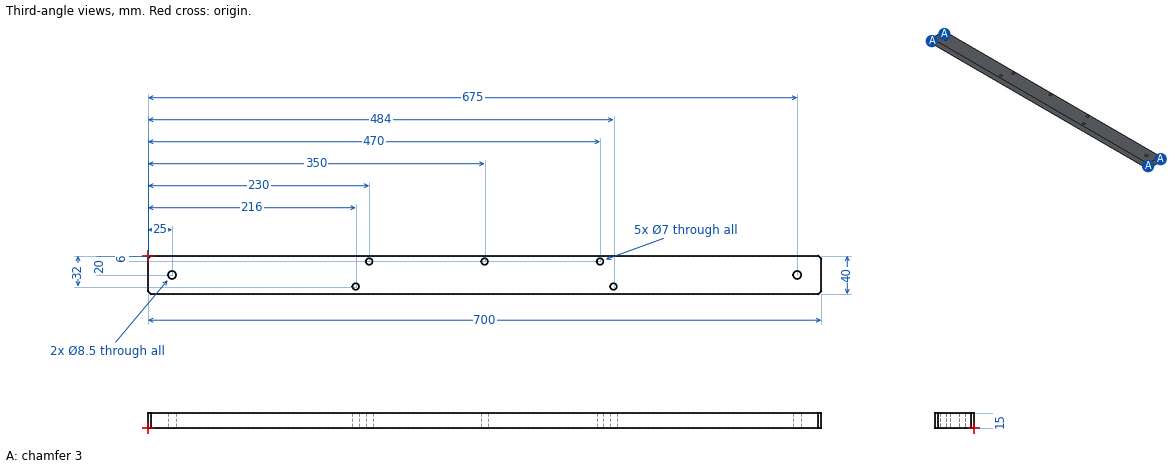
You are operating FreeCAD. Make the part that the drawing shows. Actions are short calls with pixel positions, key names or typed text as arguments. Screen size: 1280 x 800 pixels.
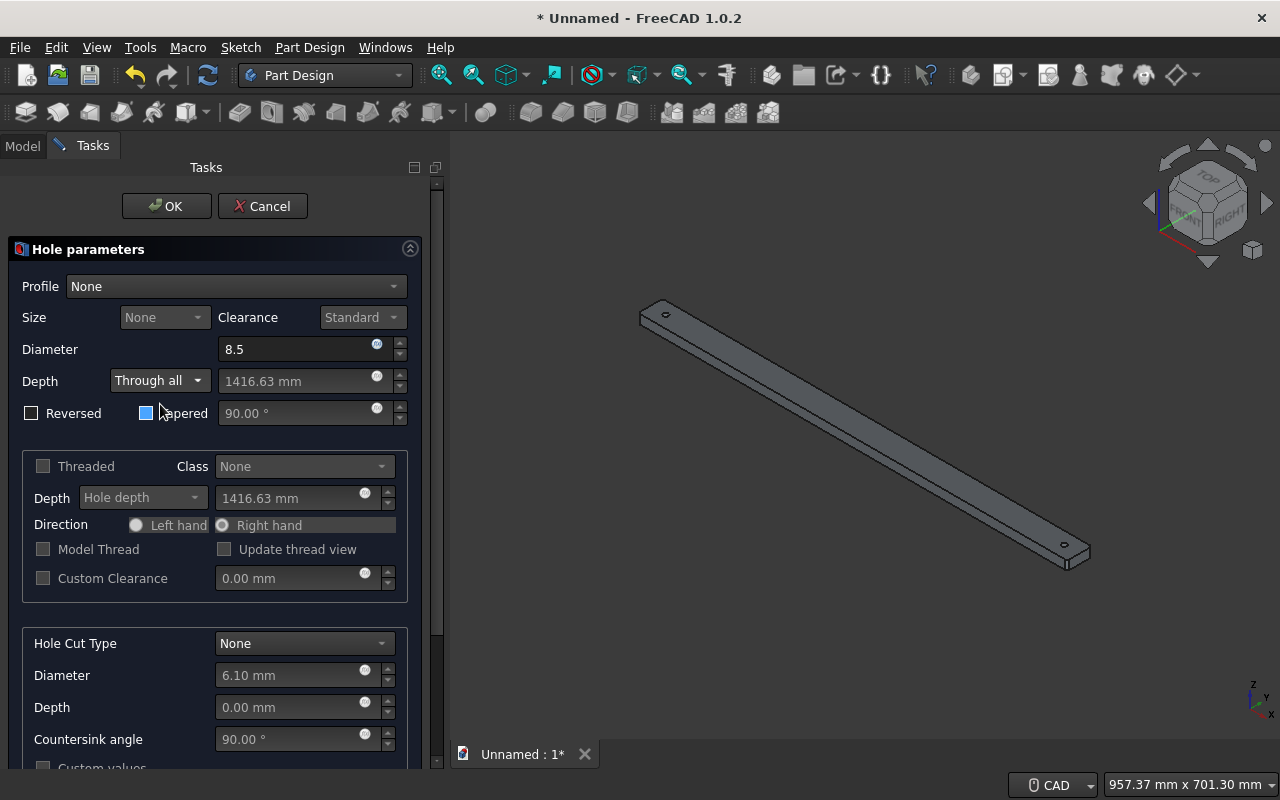
click(167, 206)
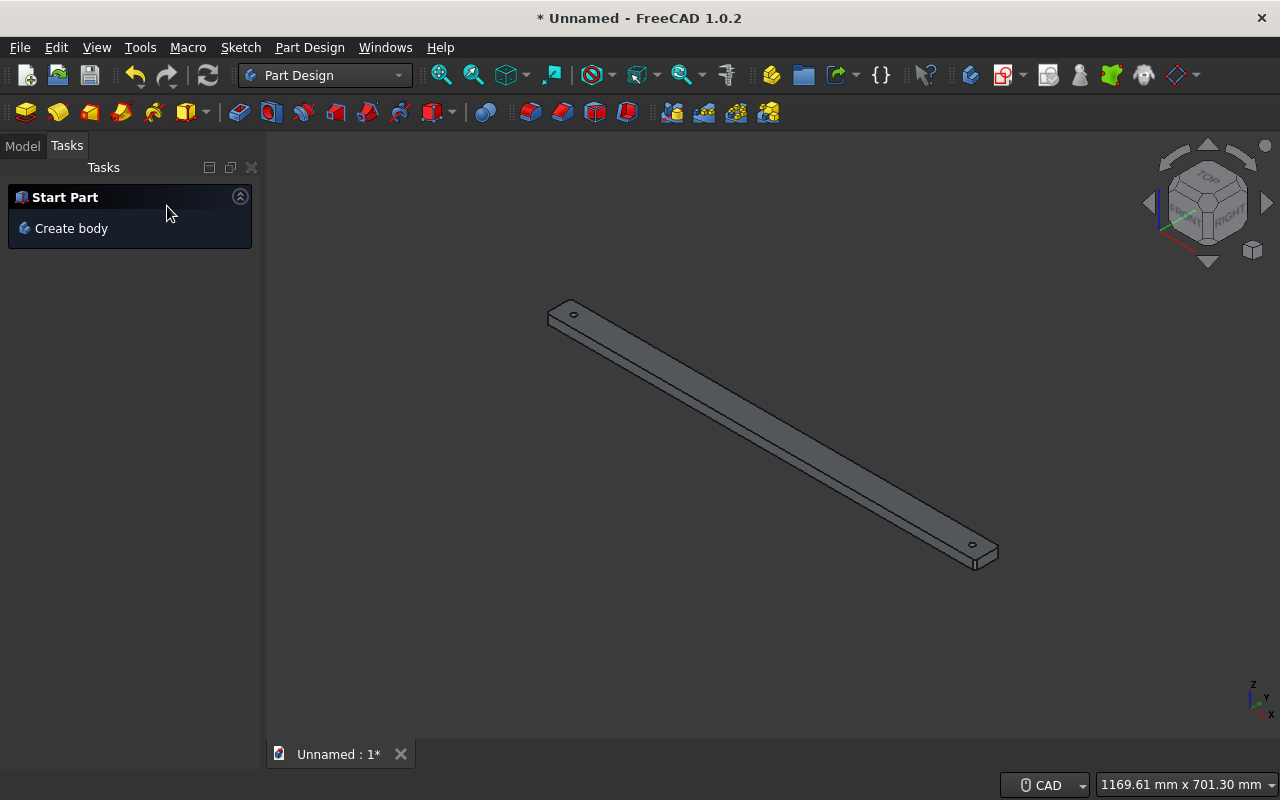
click(442, 76)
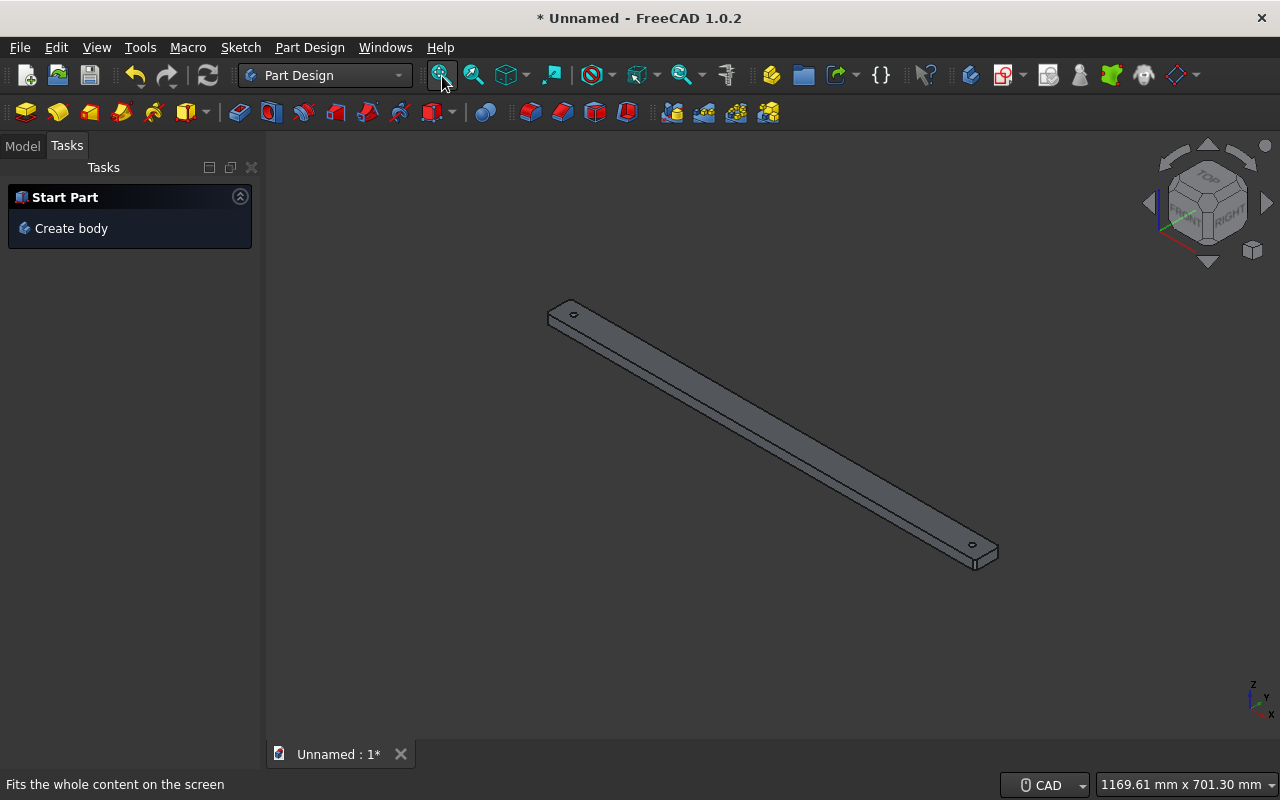
click(957, 535)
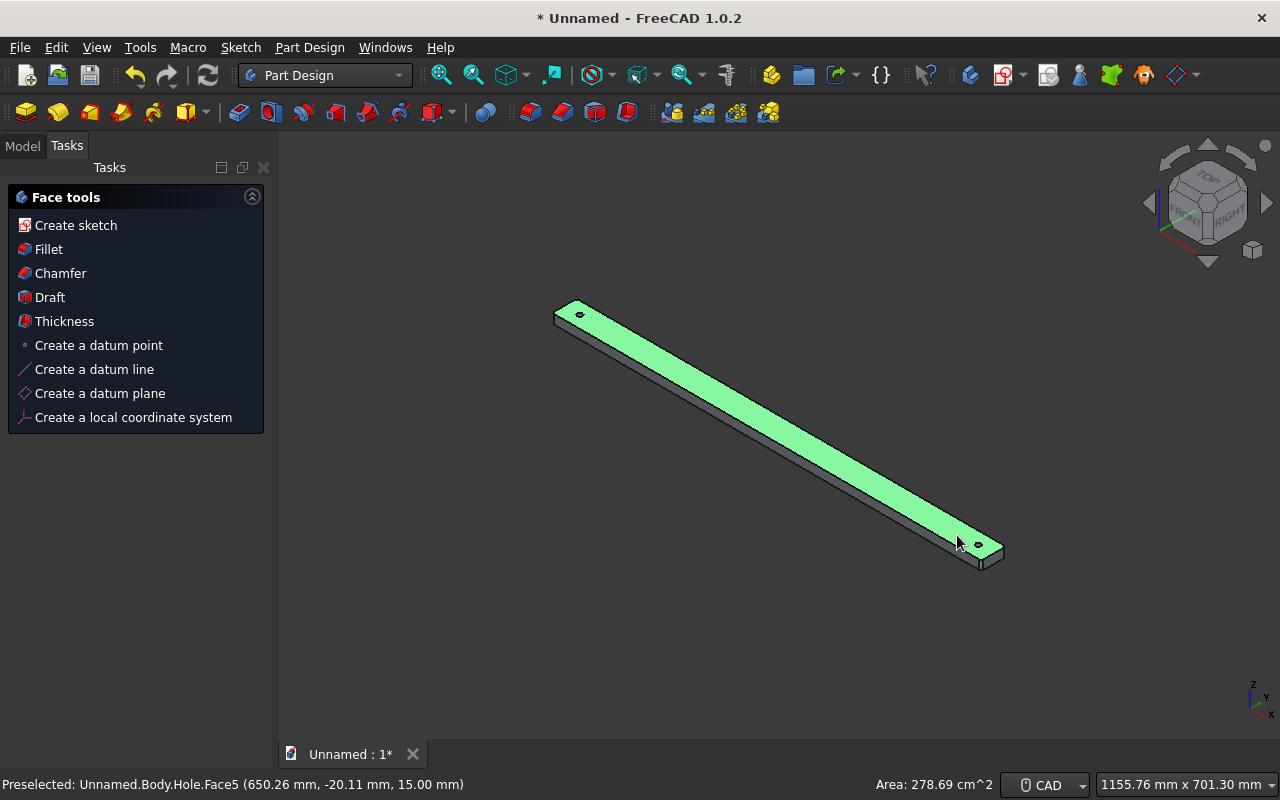
click(1004, 76)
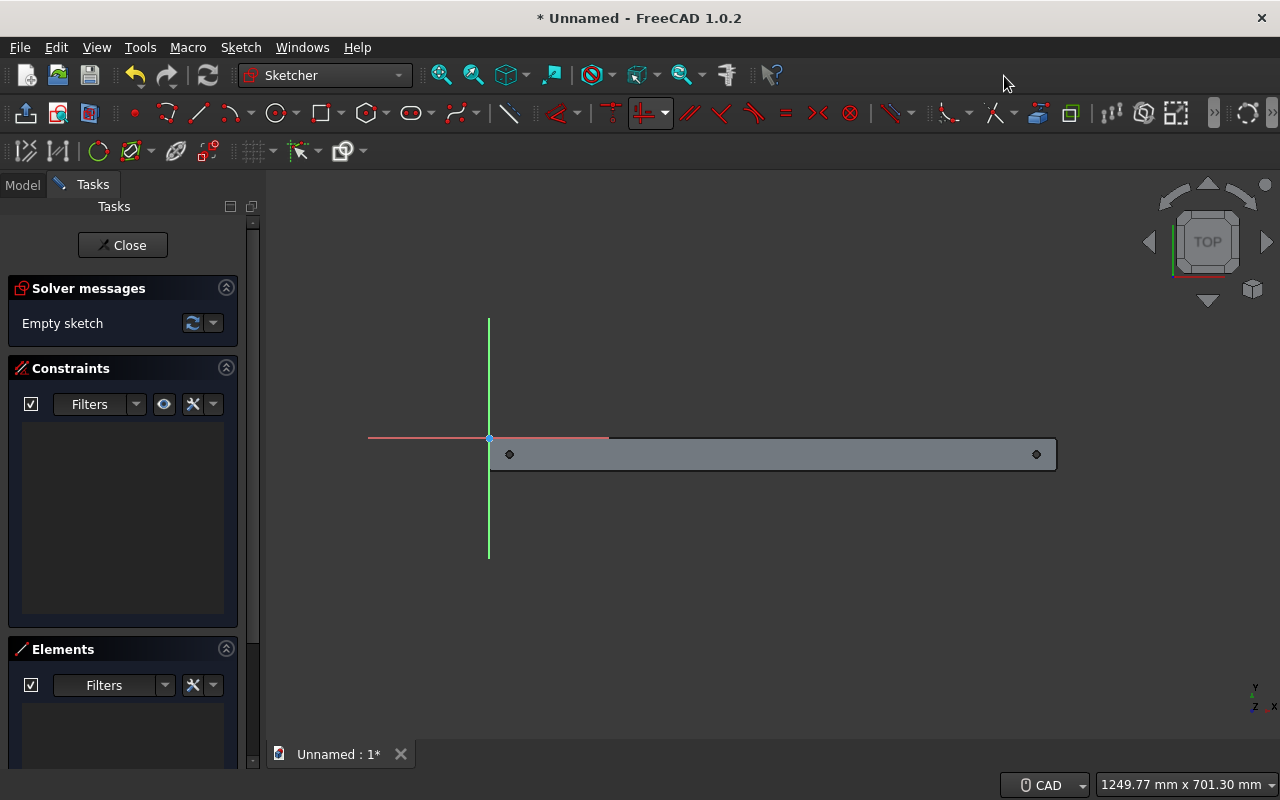
scroll(651, 449, up, 2)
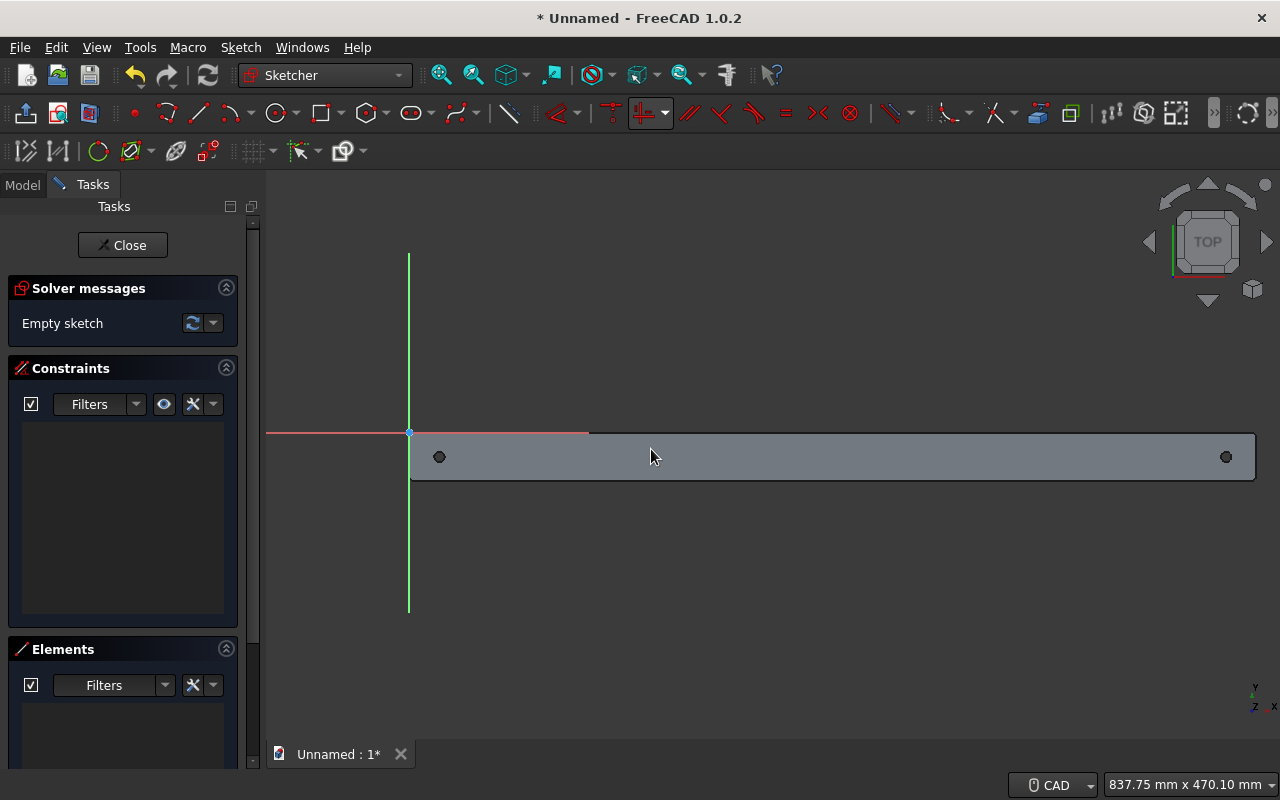
click(276, 114)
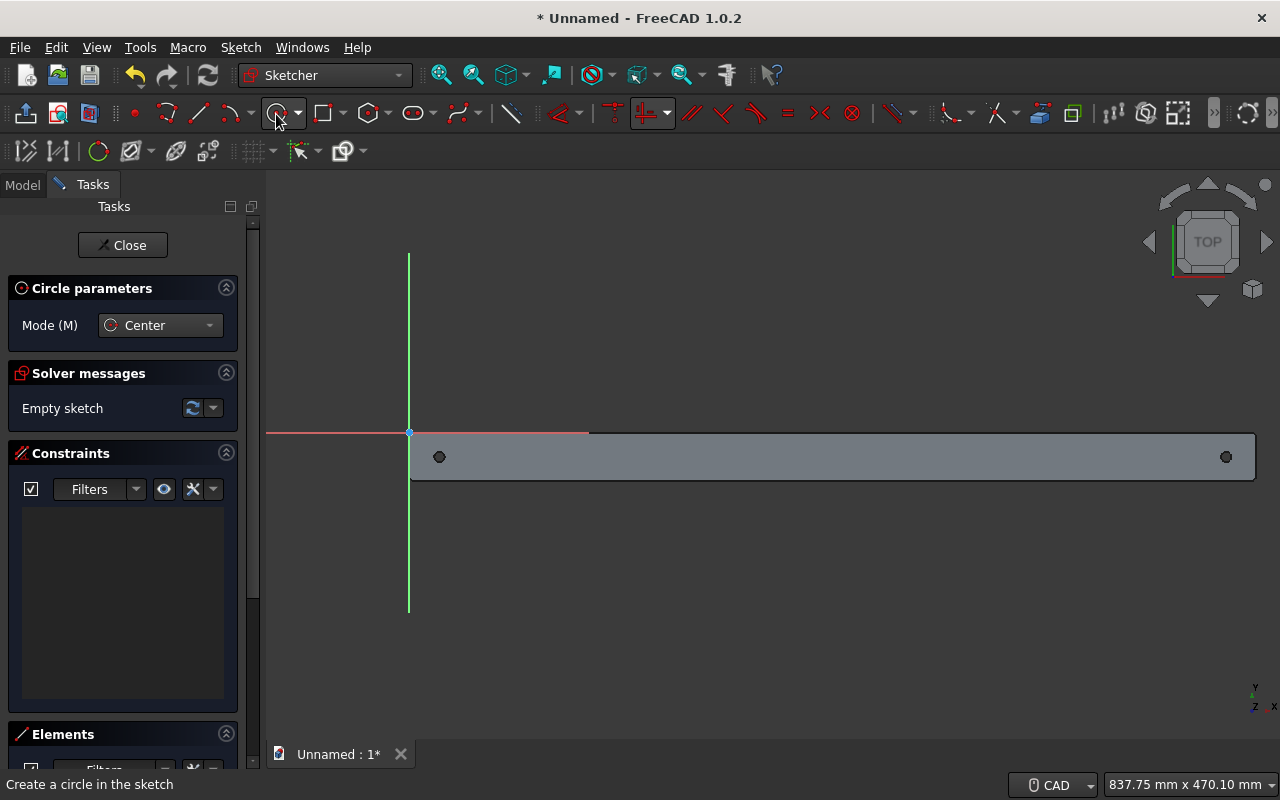
scroll(978, 440, up, 9)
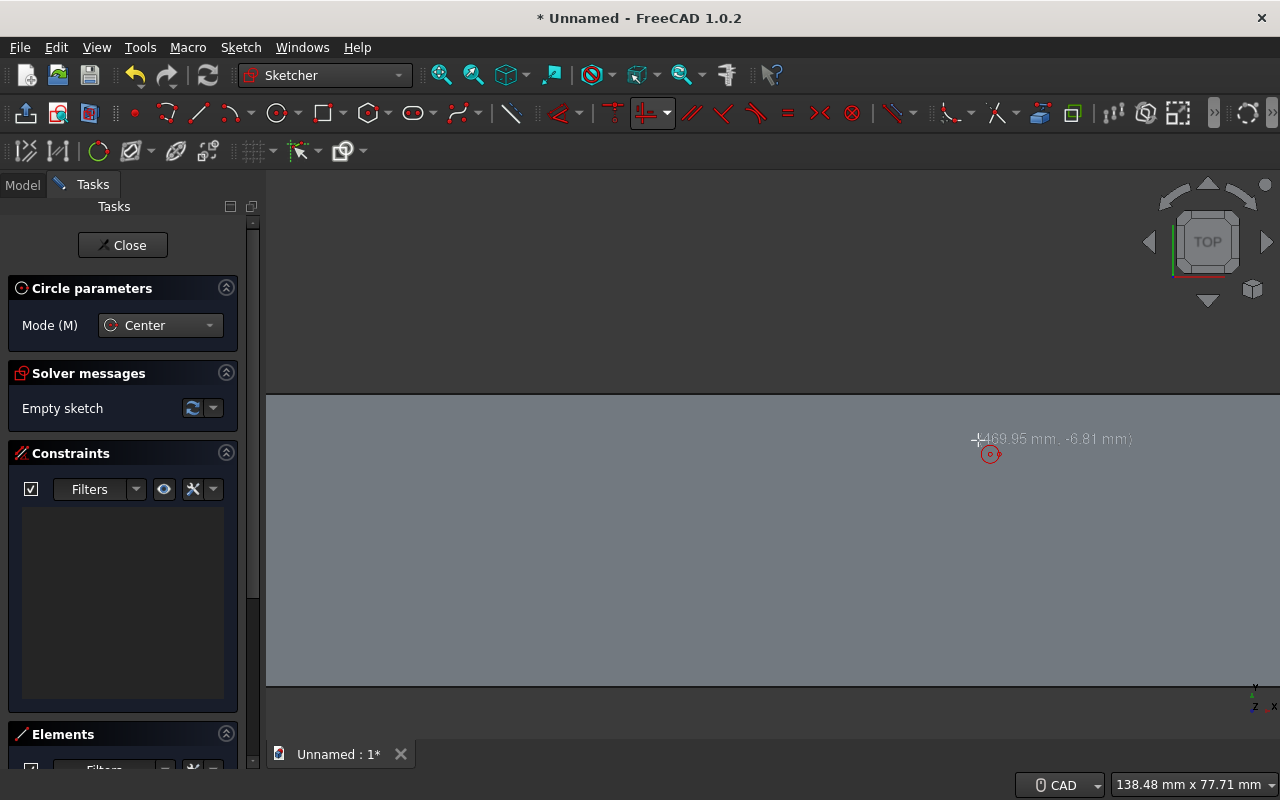
click(975, 438)
move(993, 420)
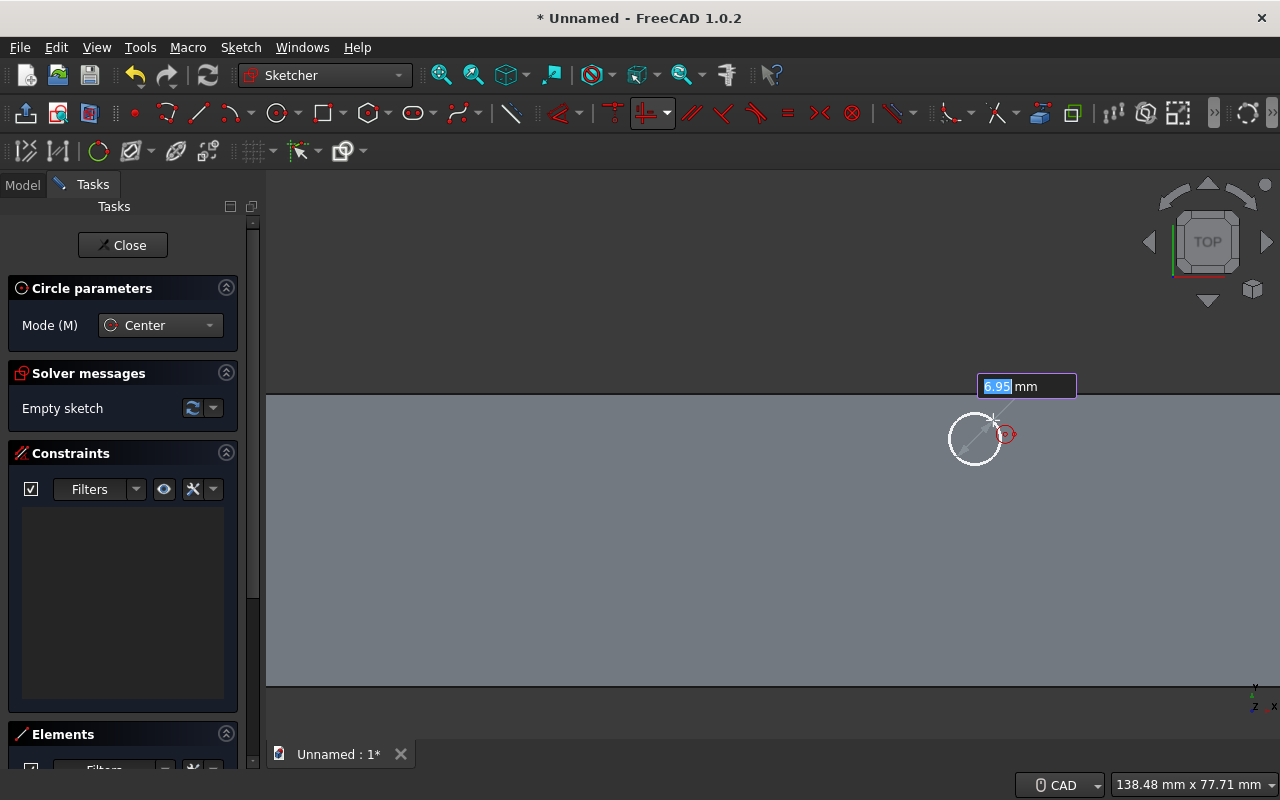
text(7)
key(Return)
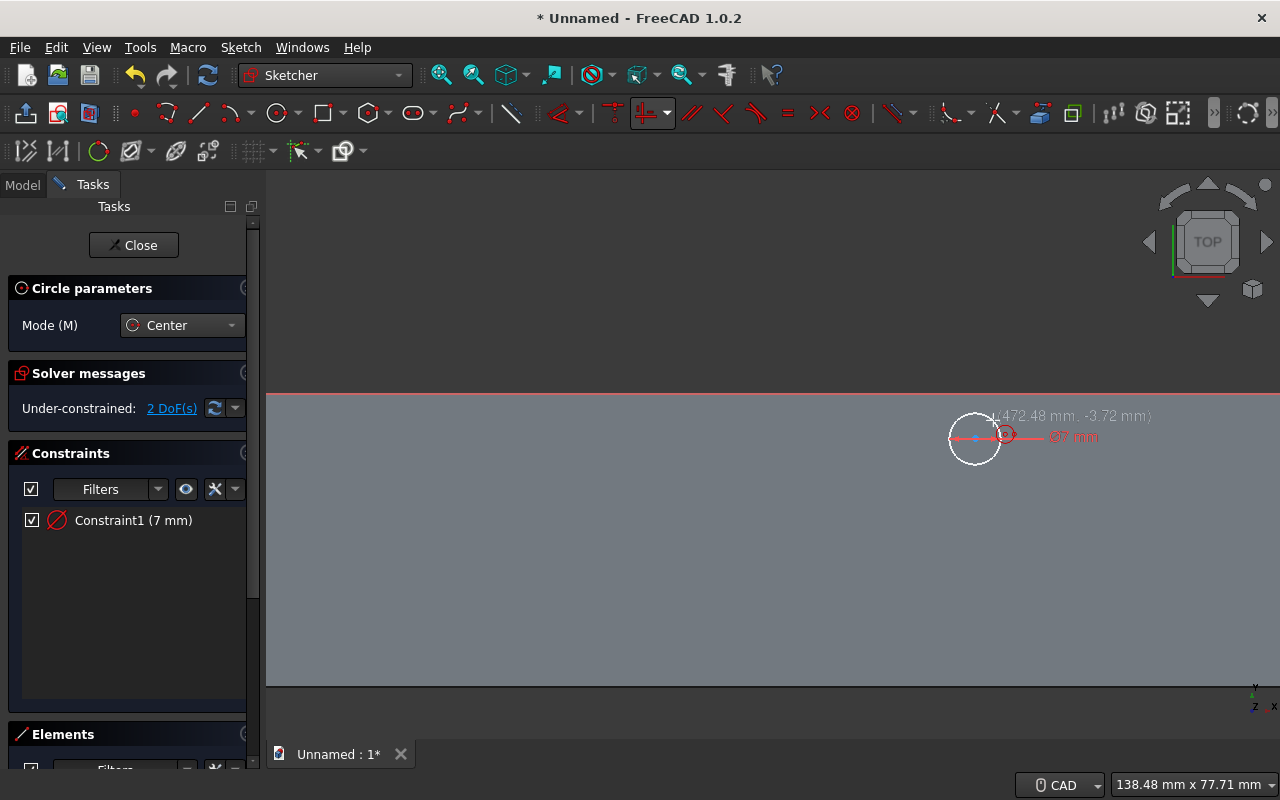
scroll(979, 441, down, 9)